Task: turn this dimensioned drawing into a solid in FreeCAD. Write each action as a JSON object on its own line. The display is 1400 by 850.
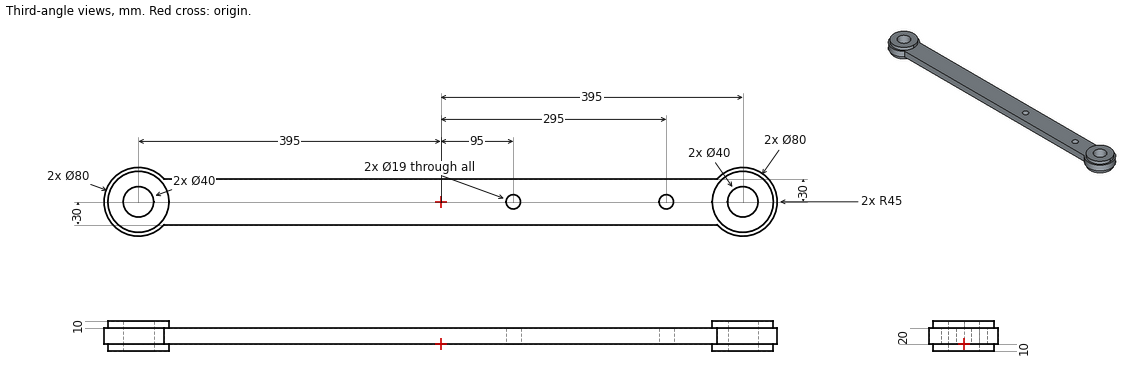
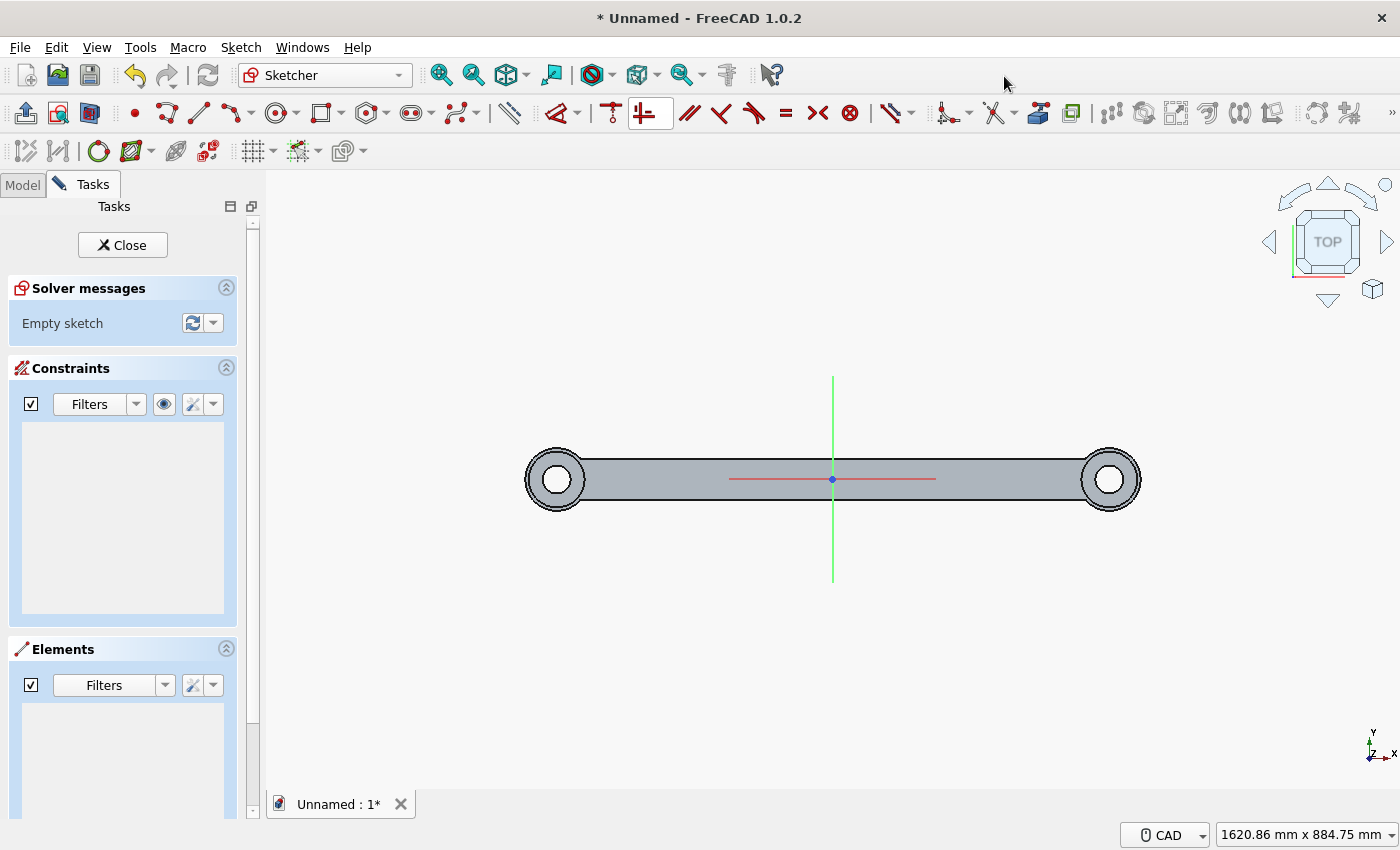
{"action": "scroll", "coordinate": [1015, 479], "scroll_direction": "up", "scroll_amount": 6}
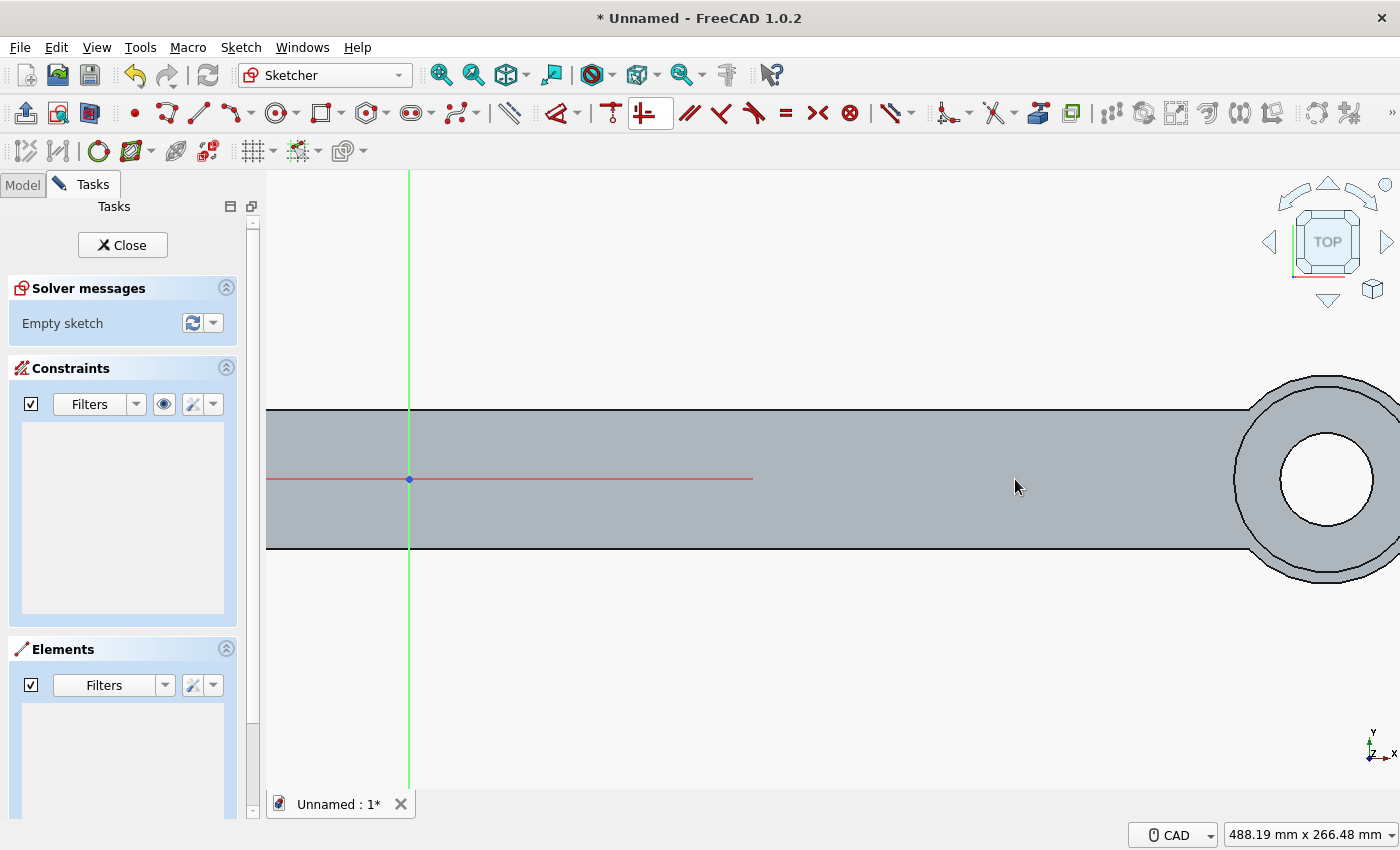
{"action": "left_click", "coordinate": [276, 114]}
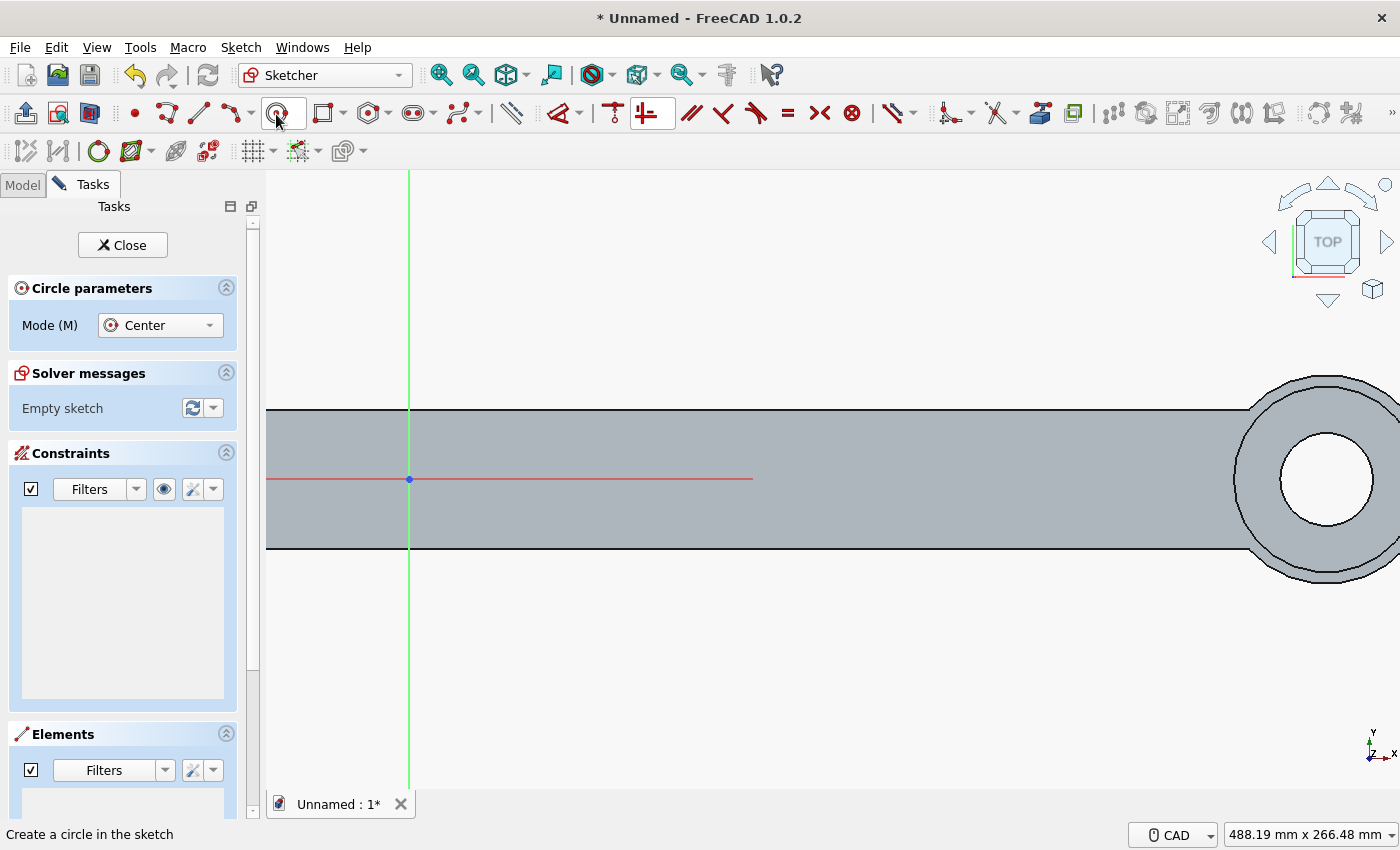
{"action": "left_click", "coordinate": [630, 479]}
{"action": "left_click", "coordinate": [645, 464]}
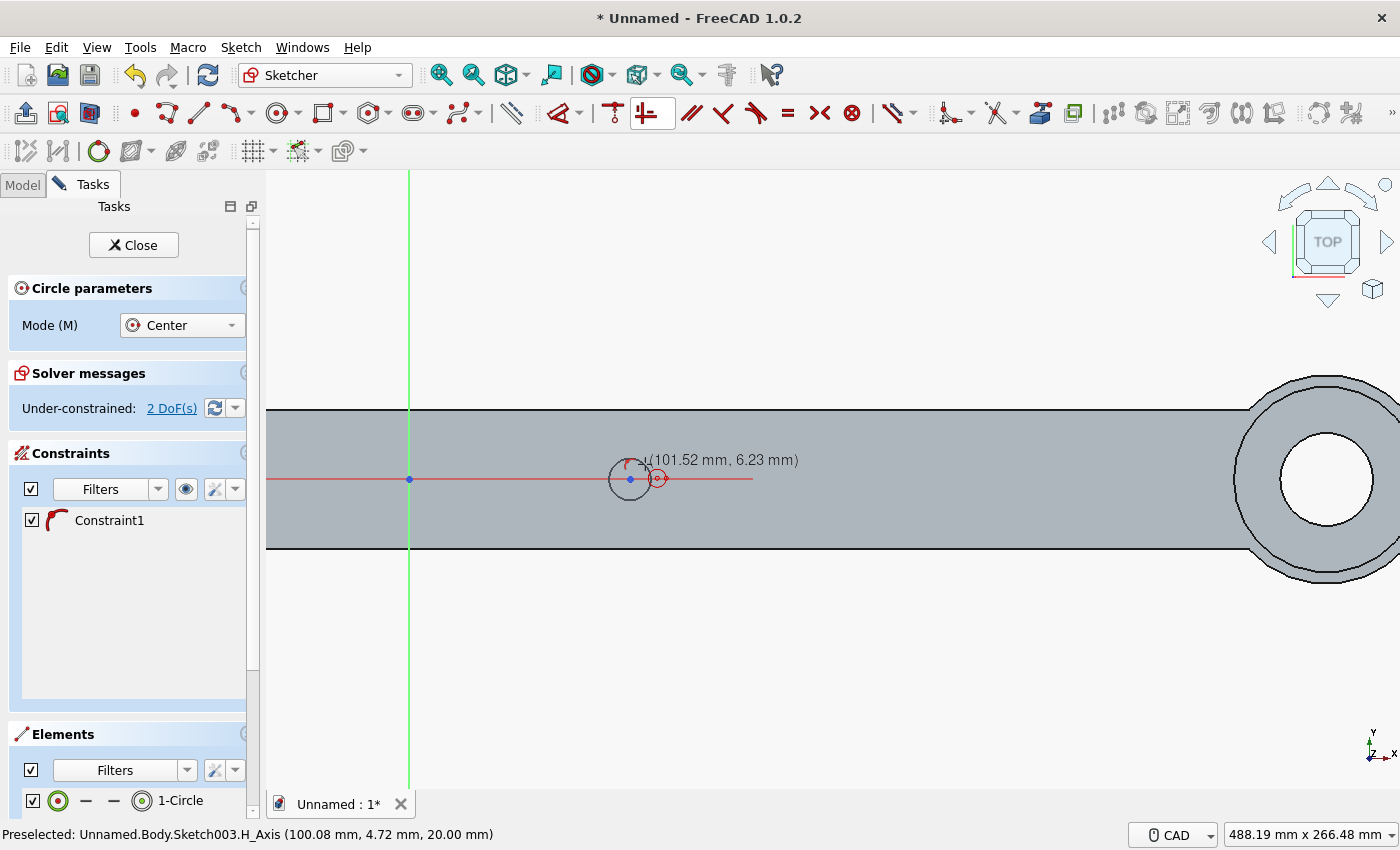
{"action": "left_click", "coordinate": [1094, 479]}
{"action": "left_click", "coordinate": [1110, 464]}
{"action": "key", "text": "Escape"}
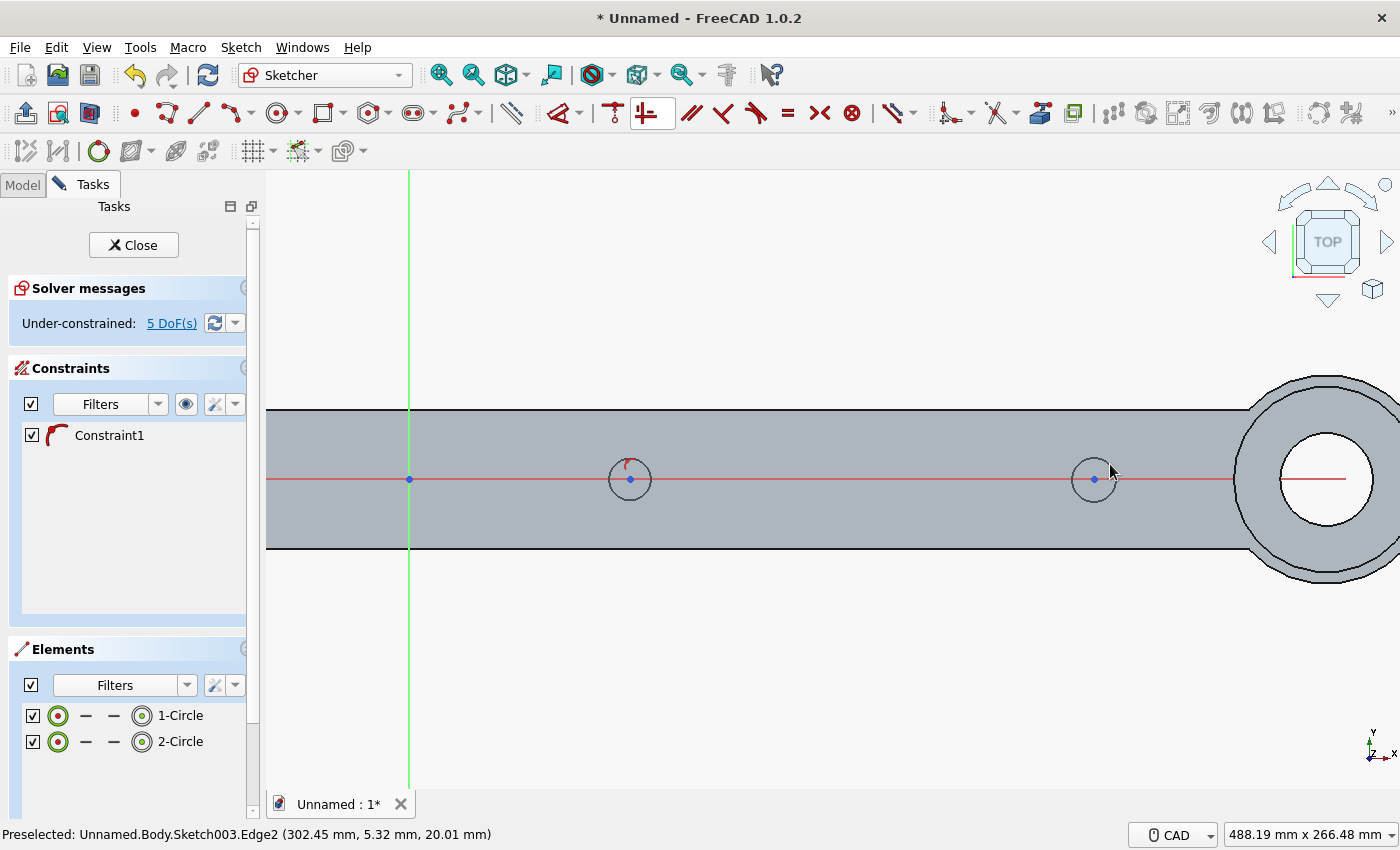
{"action": "left_click", "coordinate": [645, 465]}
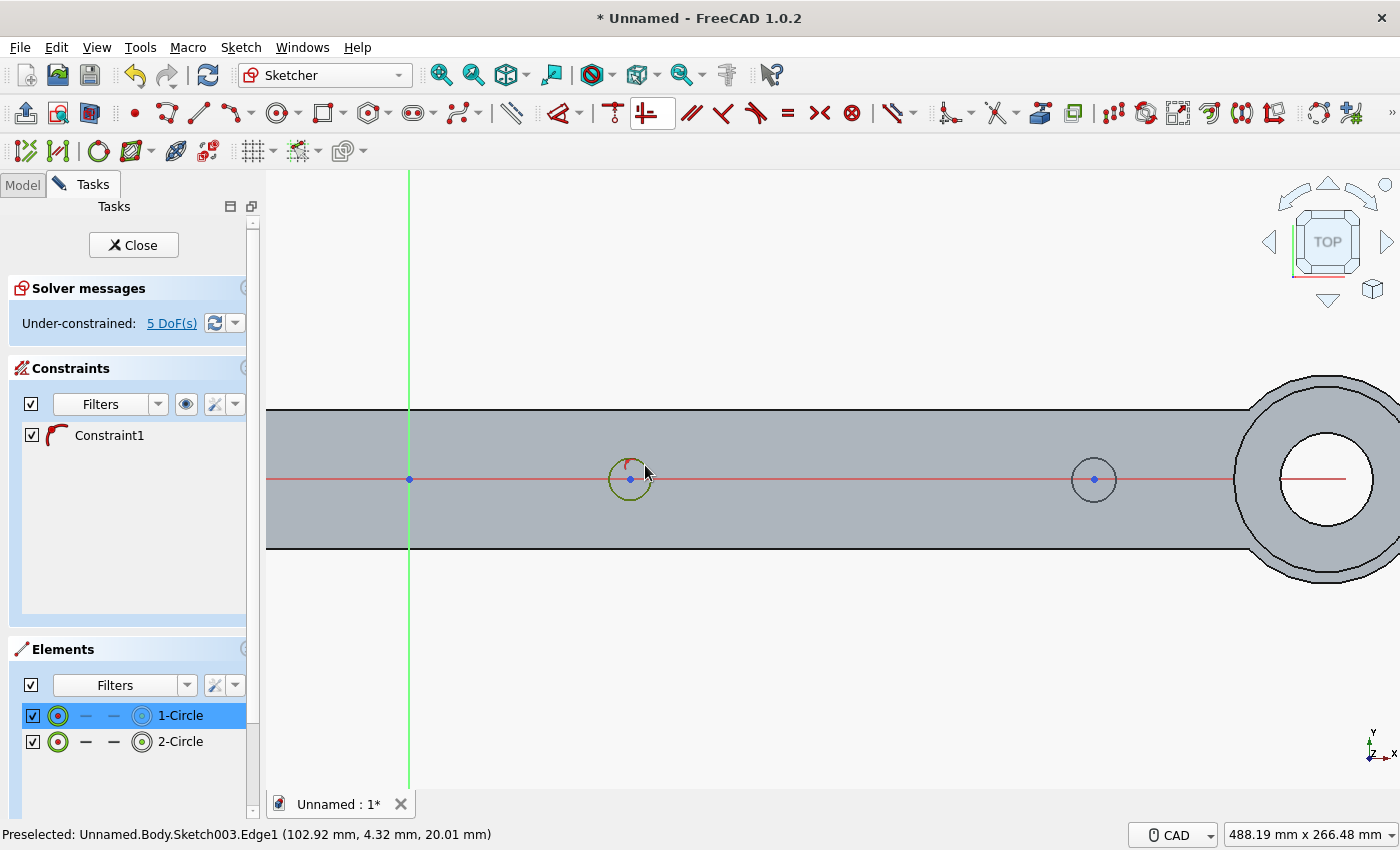
{"action": "left_click", "coordinate": [1109, 464]}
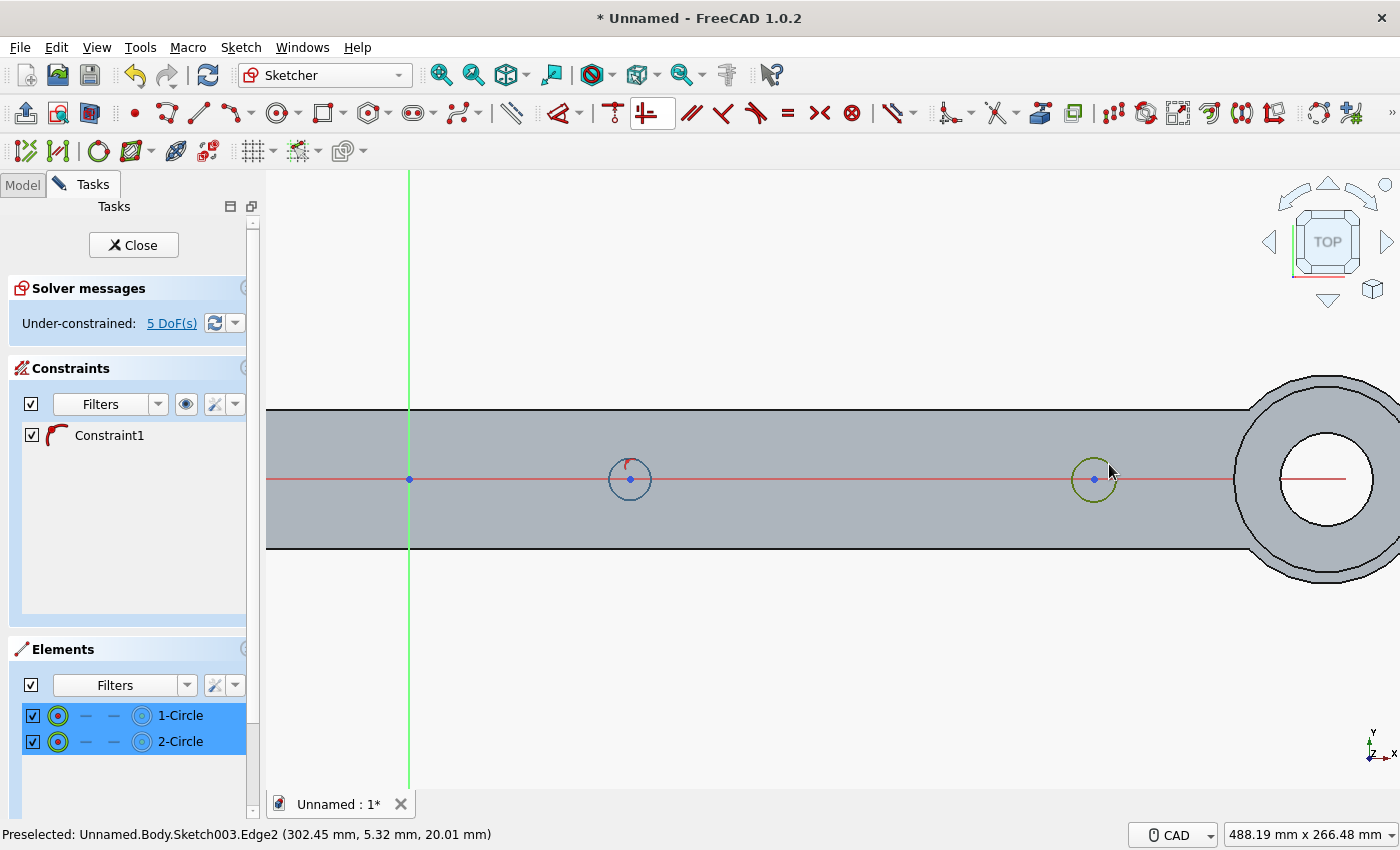
{"action": "left_click", "coordinate": [788, 114]}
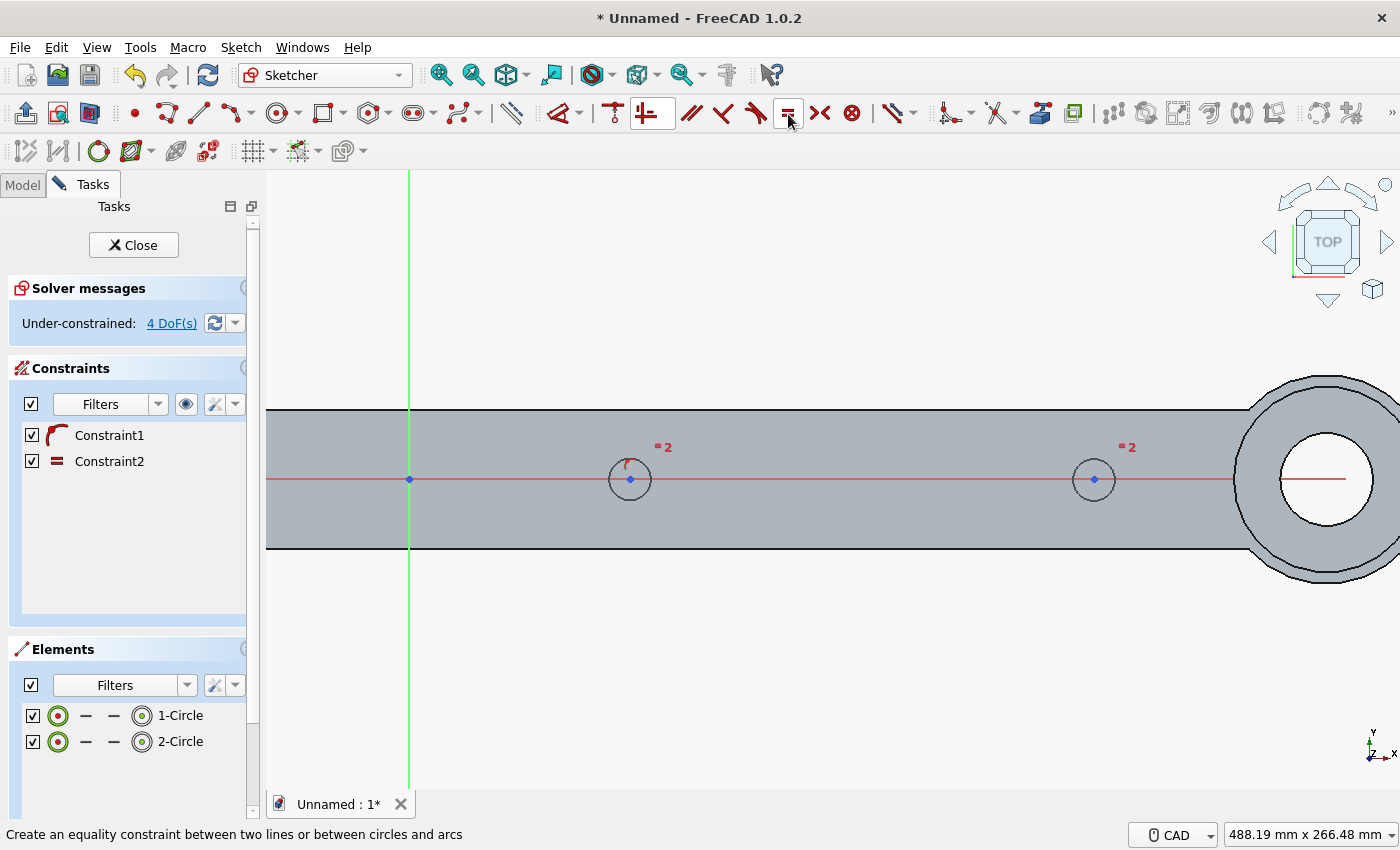
{"action": "left_click", "coordinate": [1094, 480]}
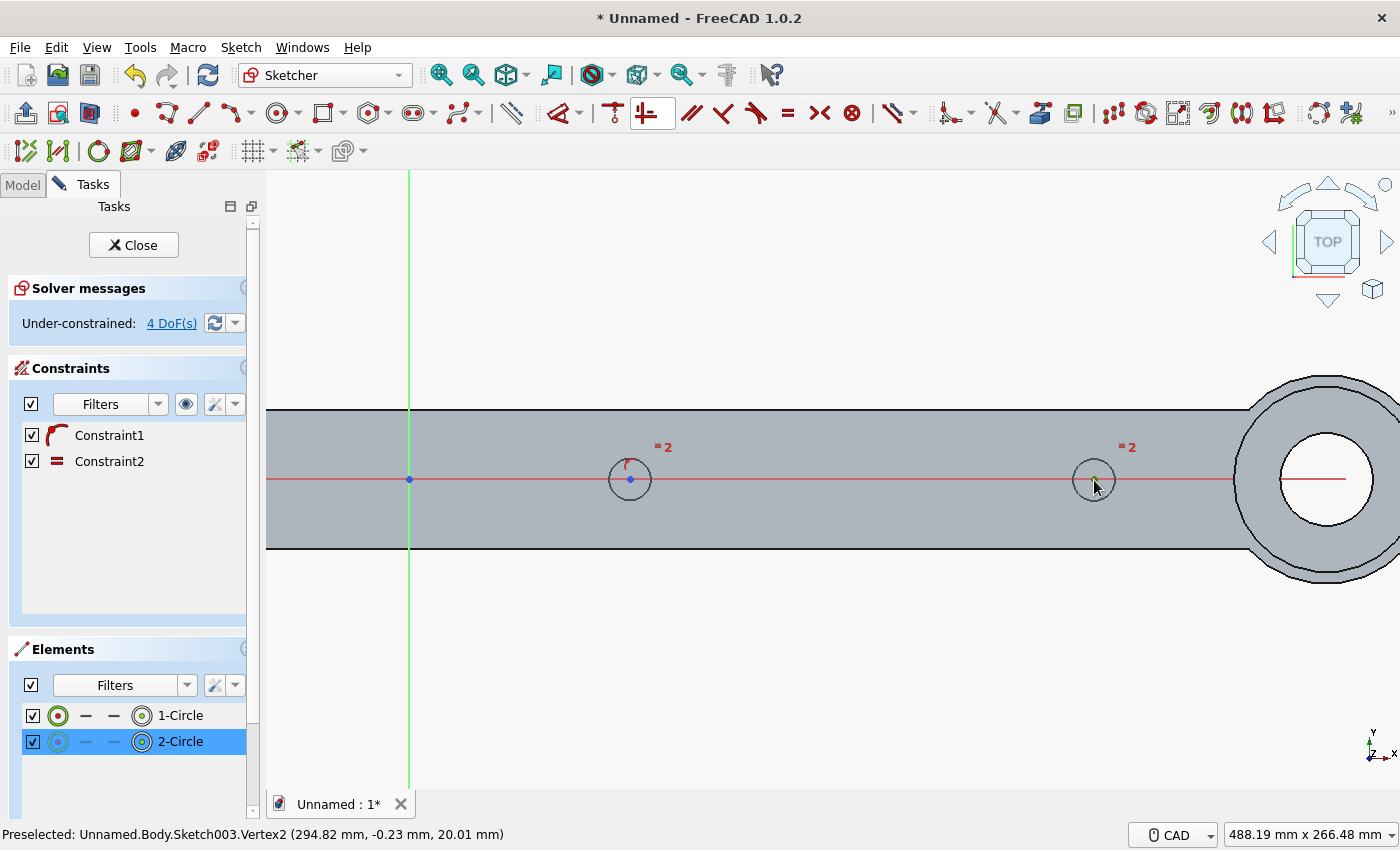
{"action": "left_click", "coordinate": [361, 479]}